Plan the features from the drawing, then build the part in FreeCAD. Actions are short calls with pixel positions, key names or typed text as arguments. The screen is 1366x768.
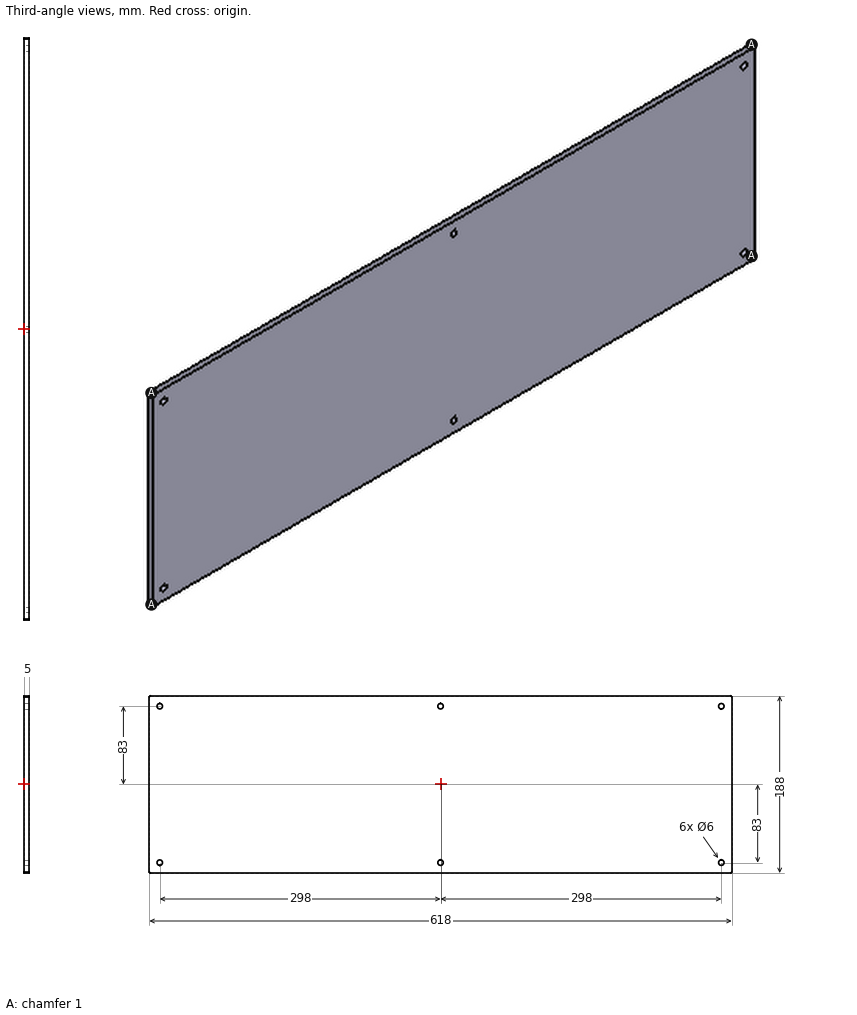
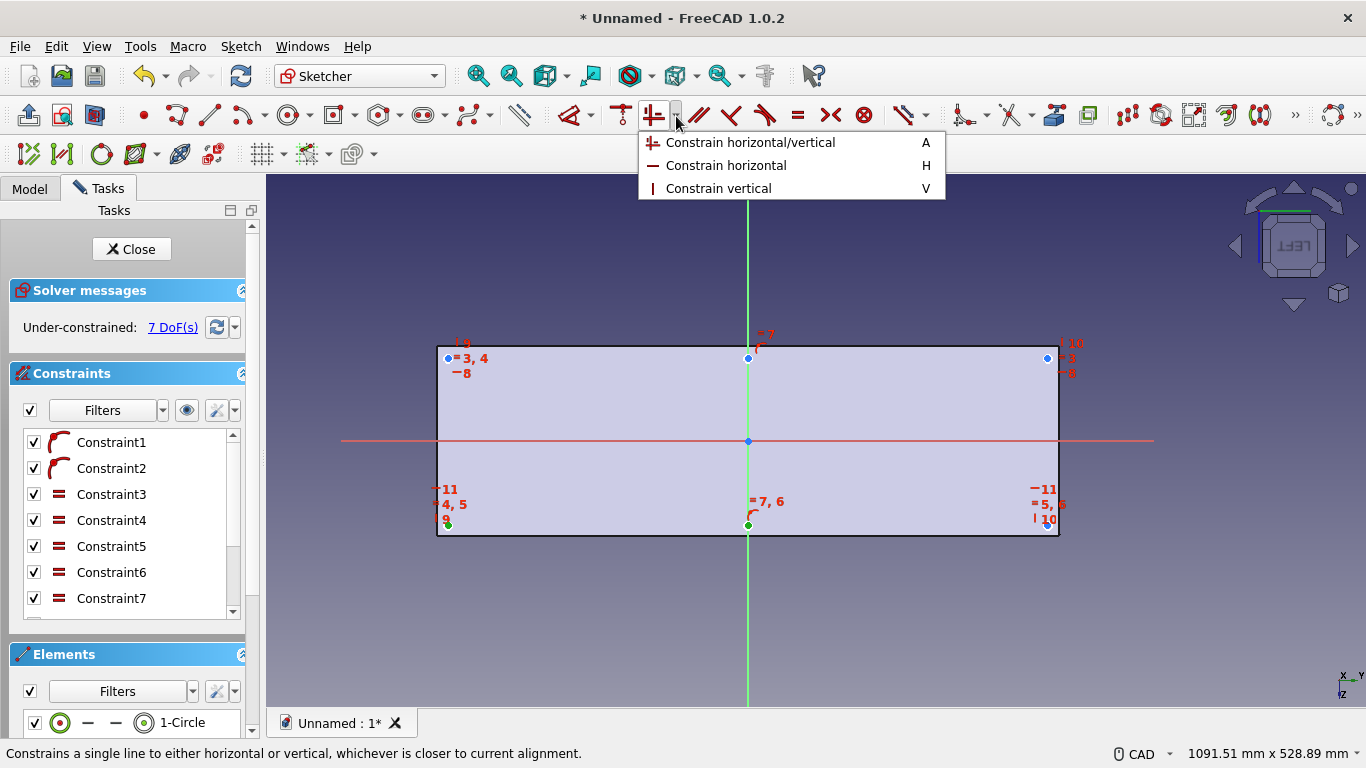
click(792, 166)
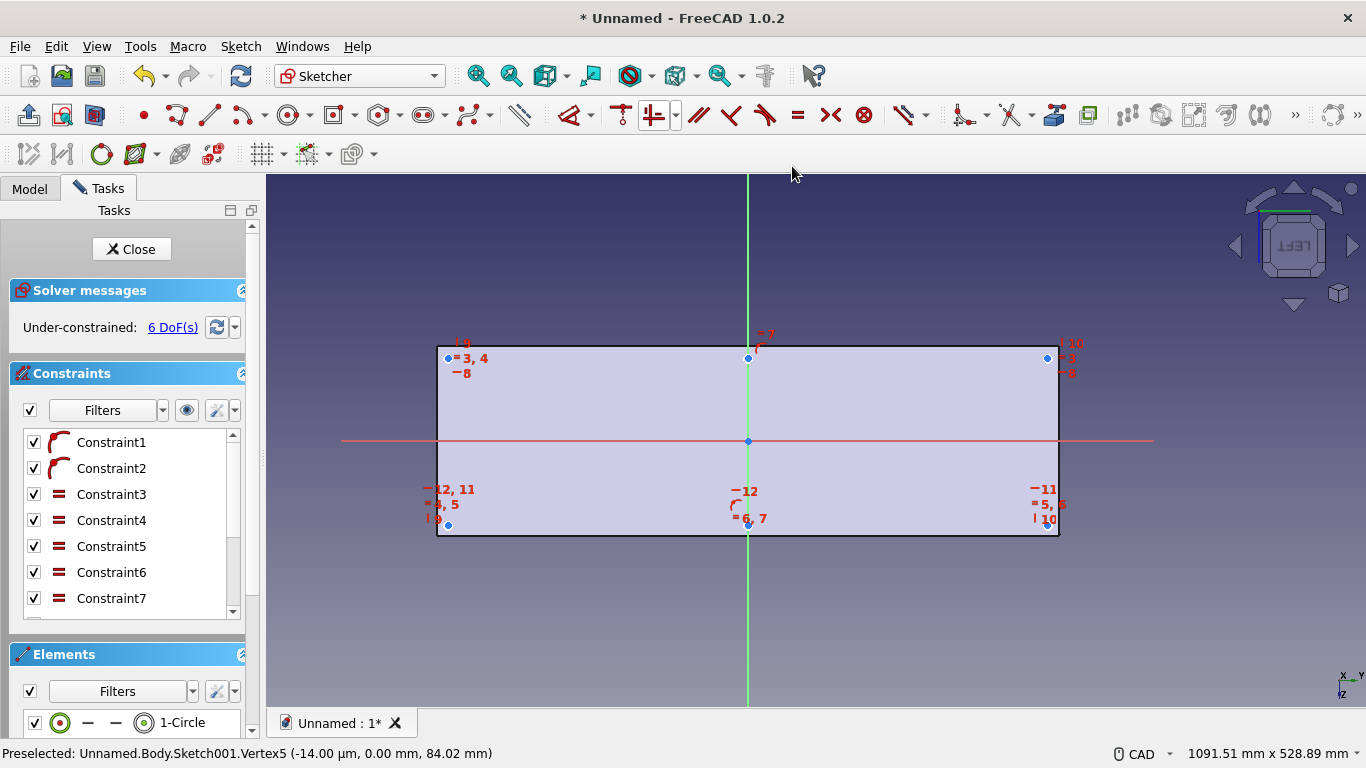
click(1048, 359)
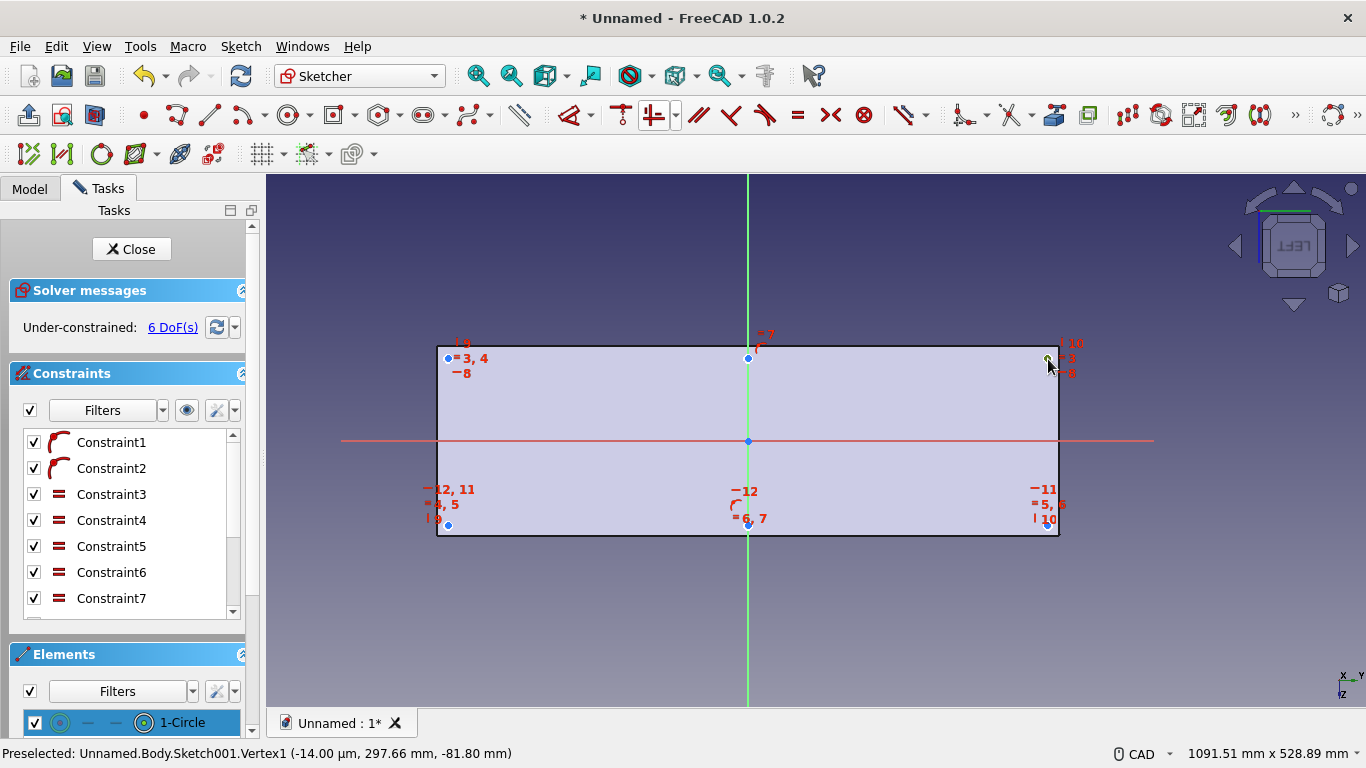
click(748, 359)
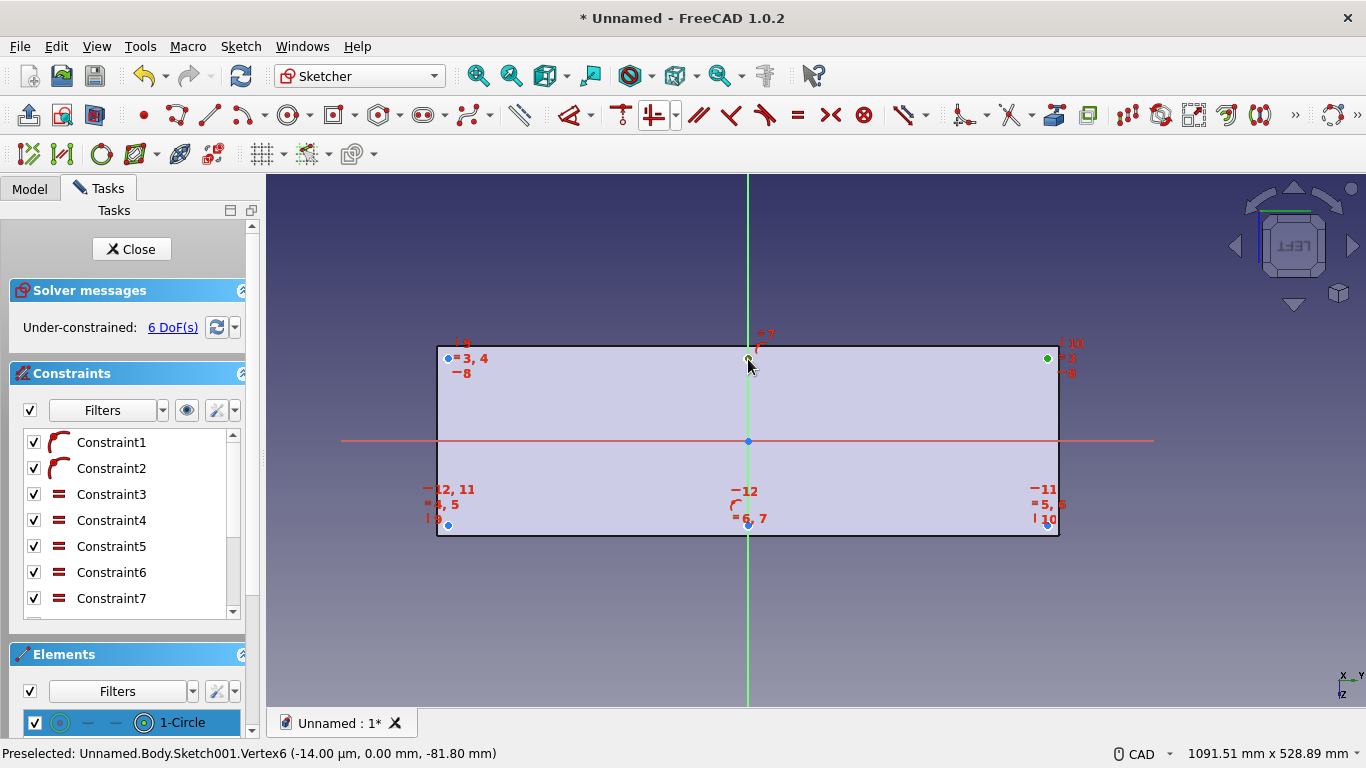
click(676, 116)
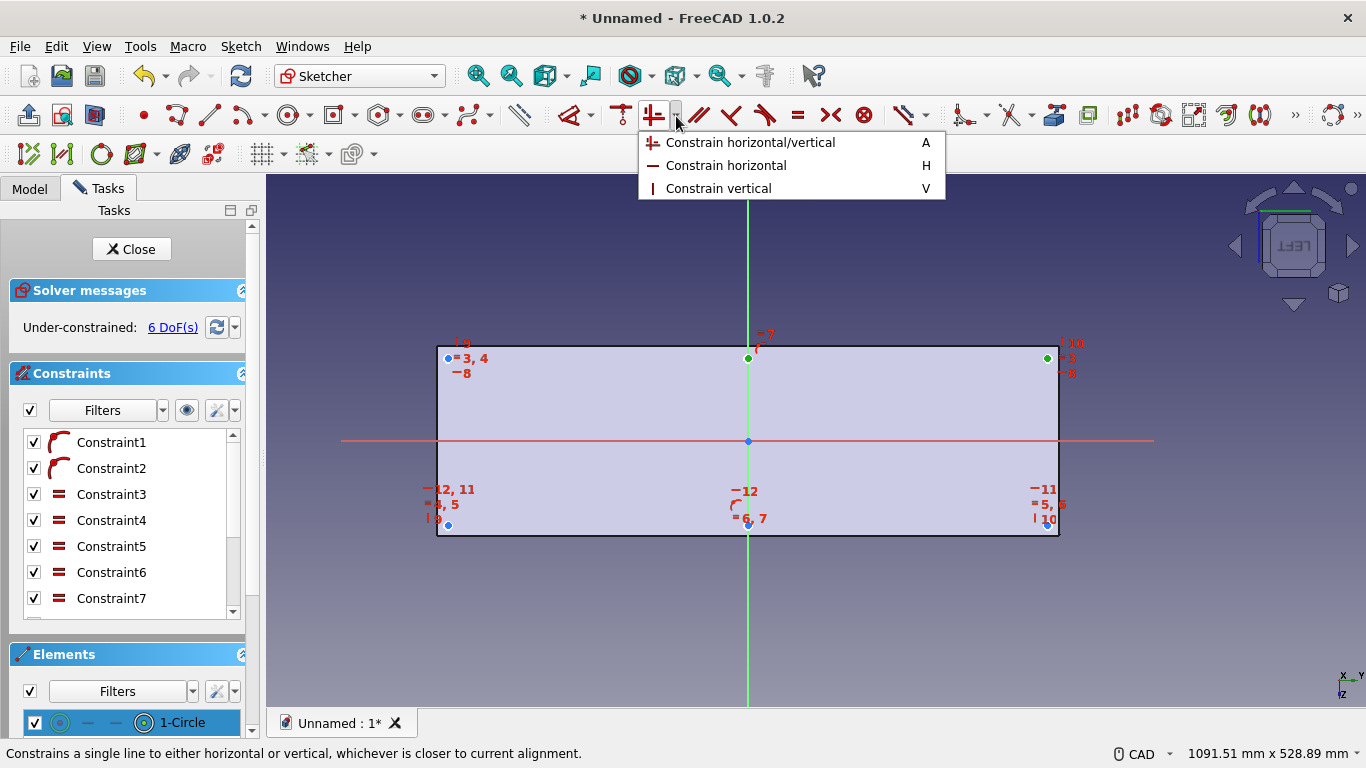
click(792, 166)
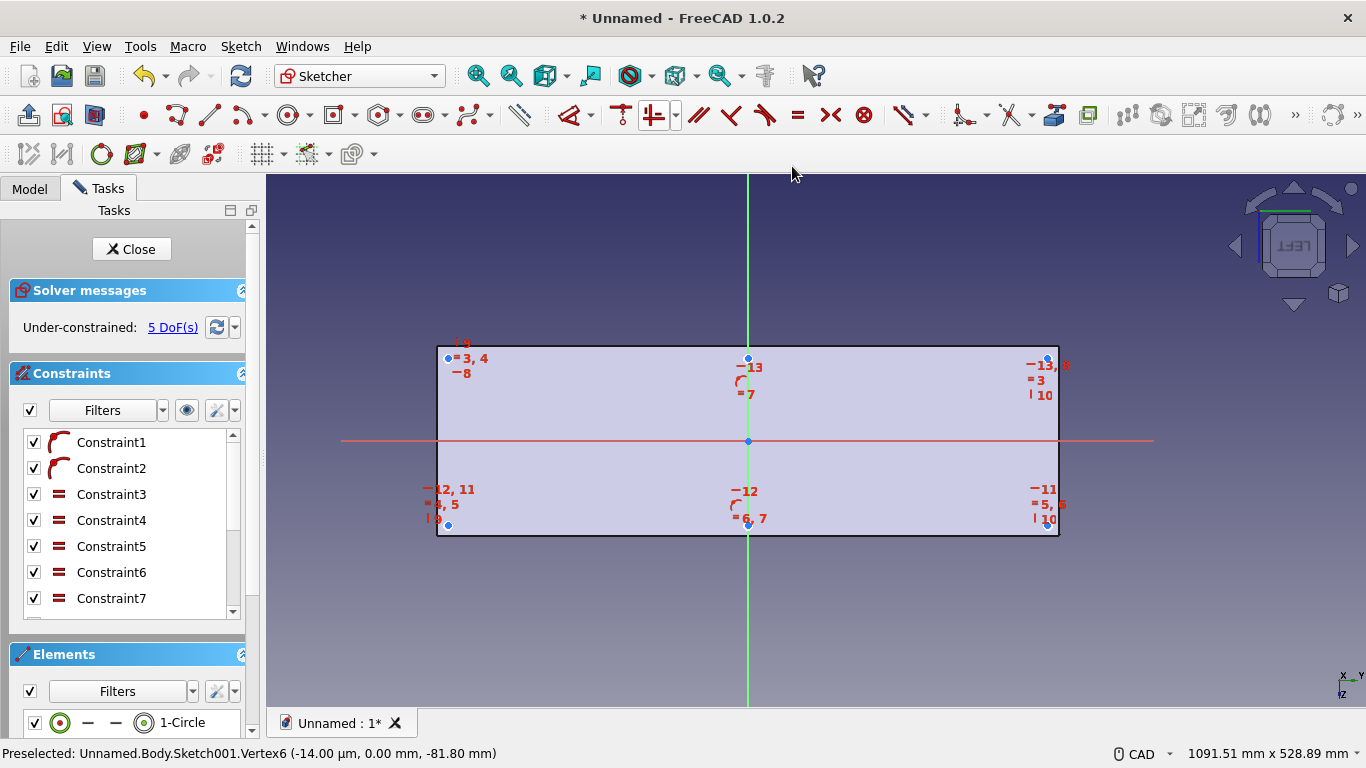
click(568, 116)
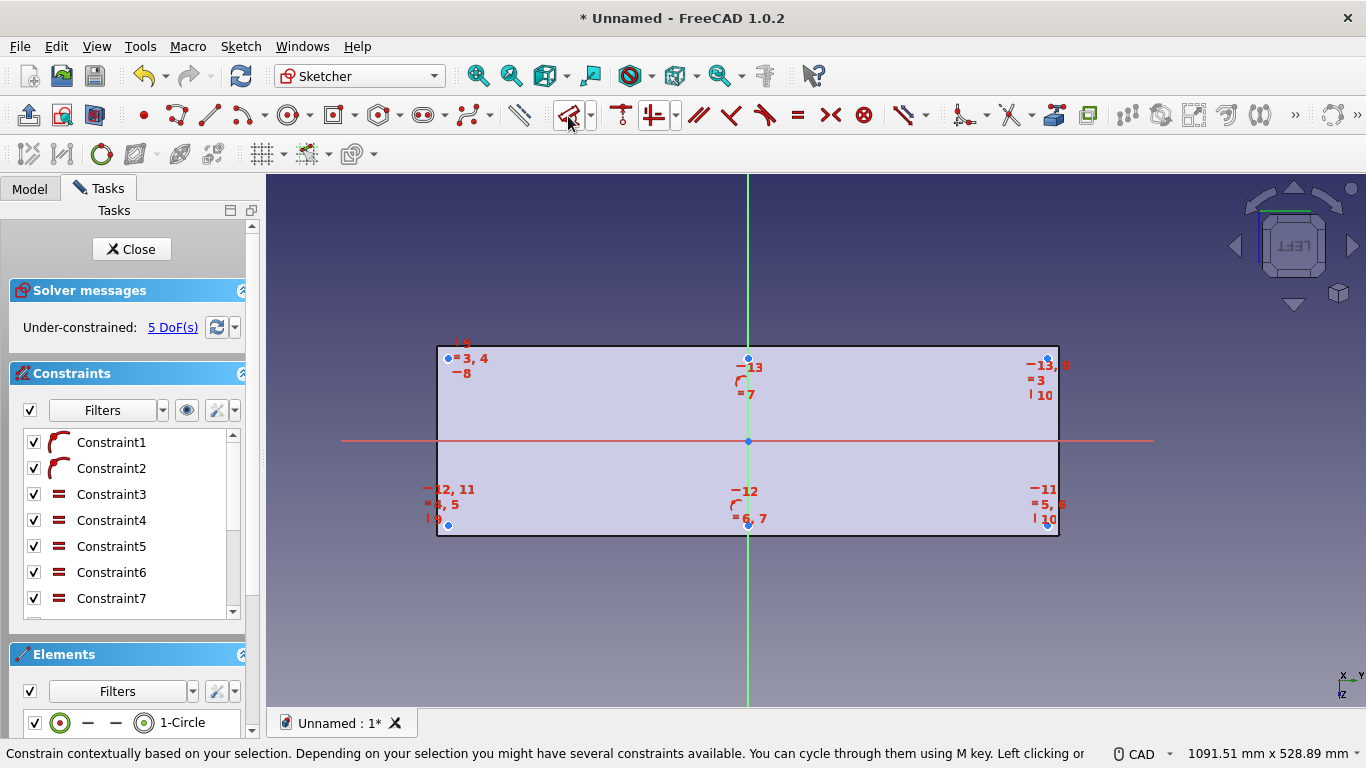
scroll(1051, 356, up, 10)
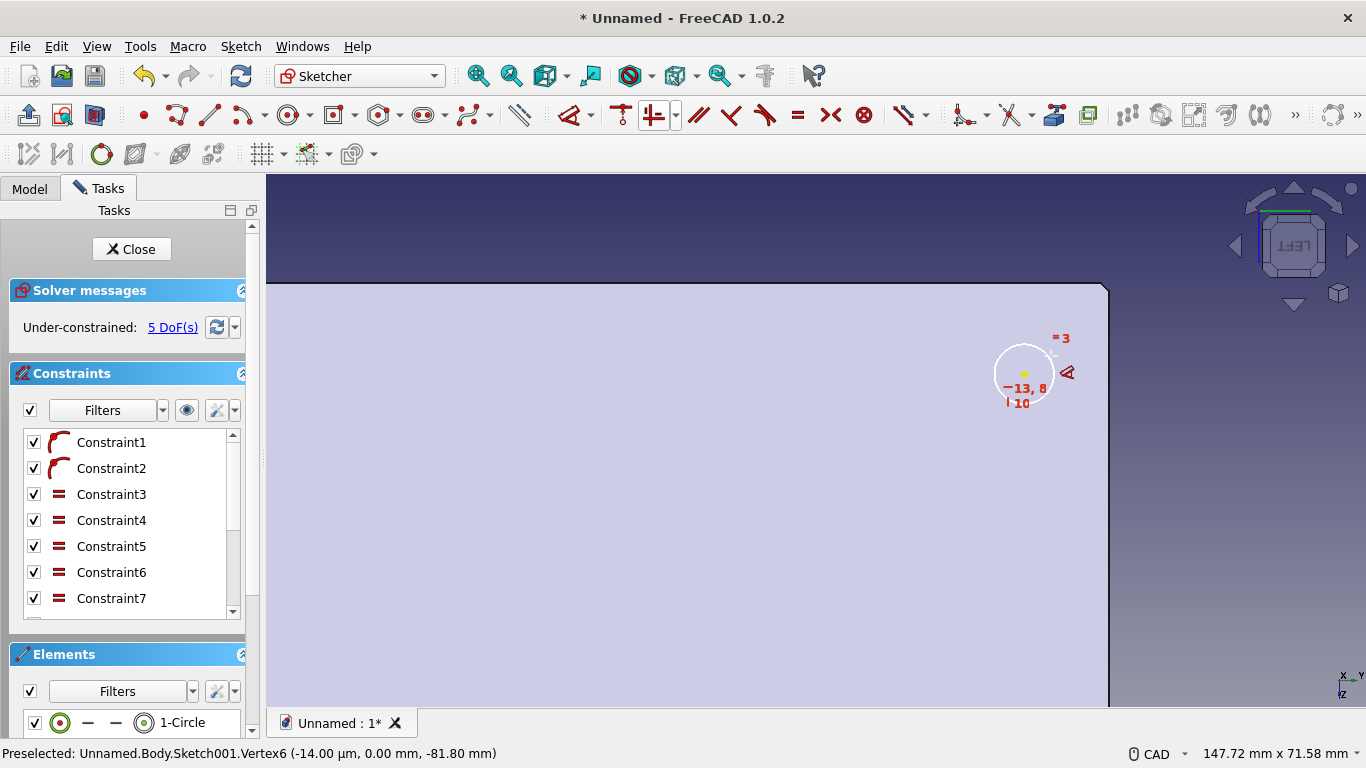
click(1045, 353)
click(1067, 330)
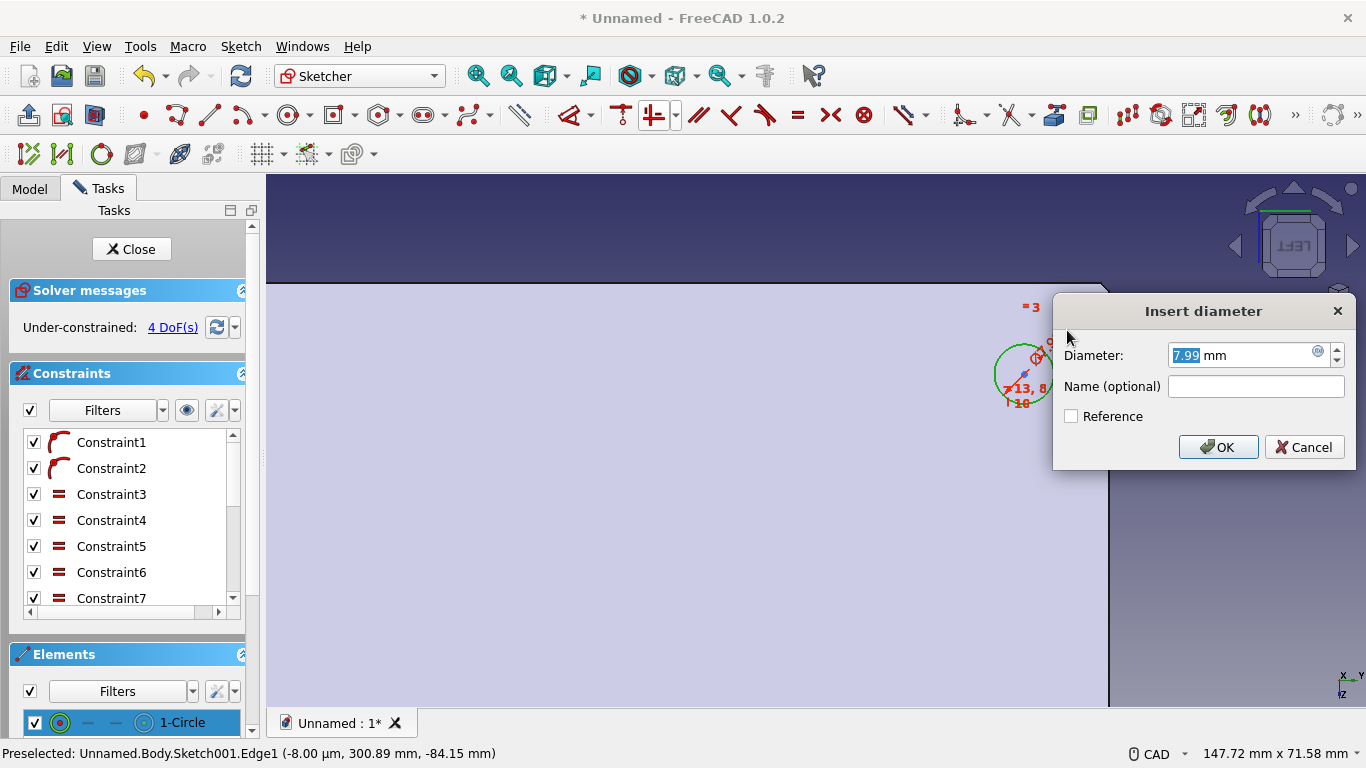
text(6)
key(Return)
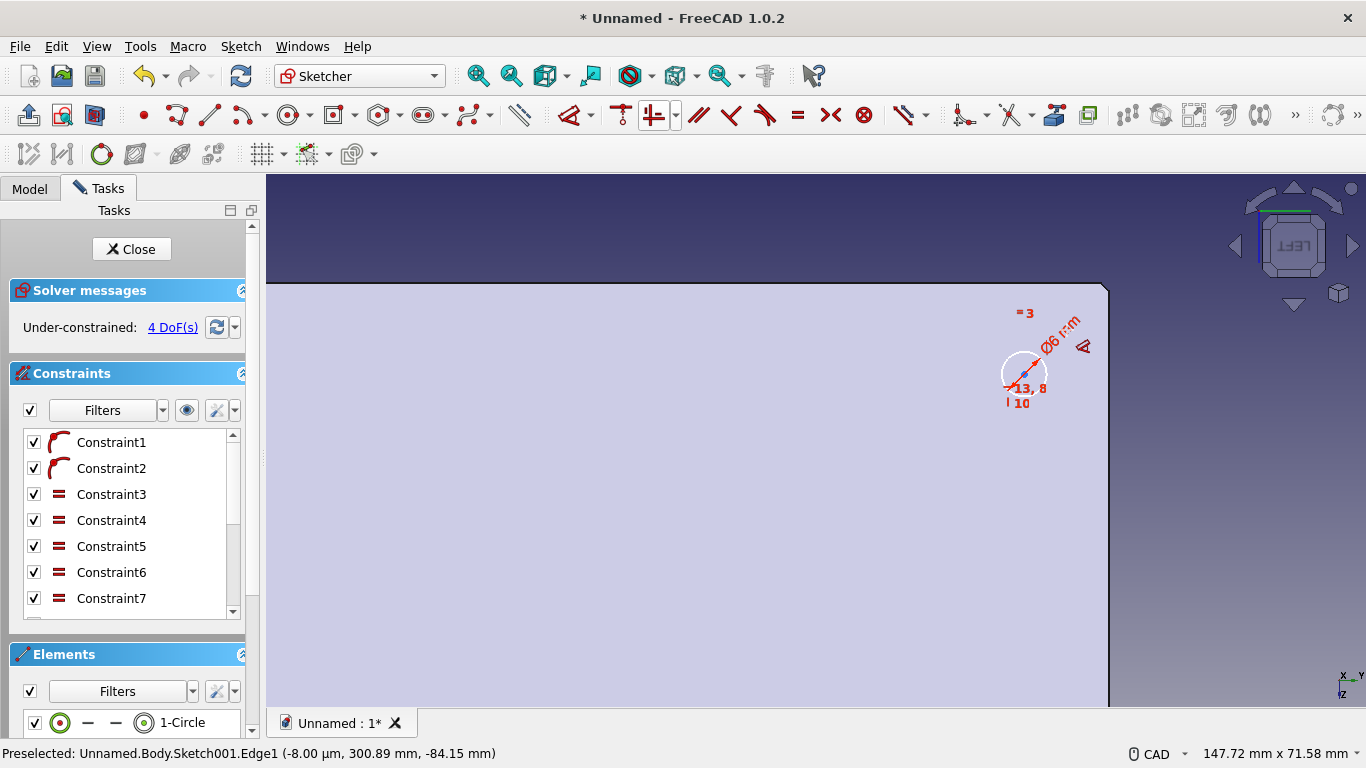
scroll(1051, 356, down, 10)